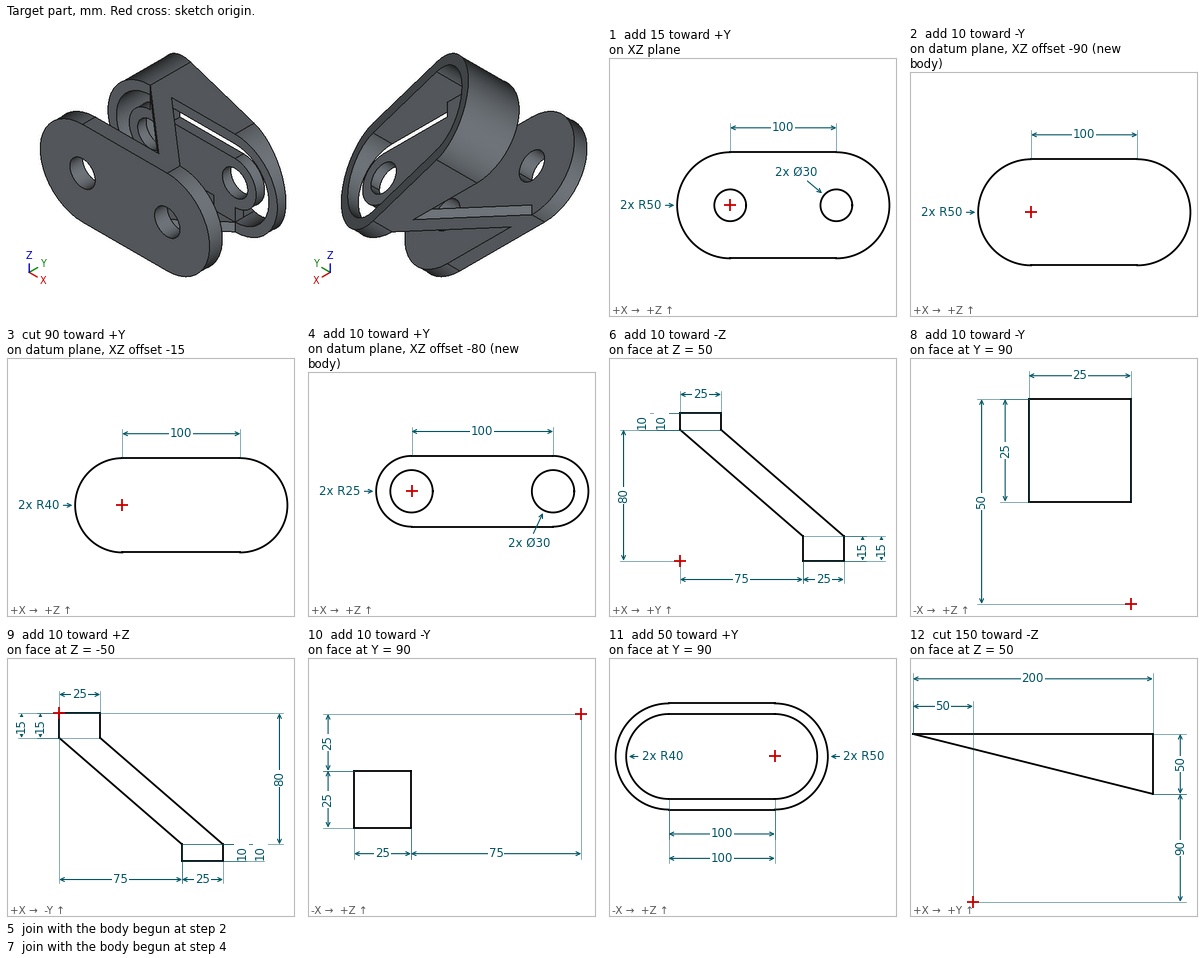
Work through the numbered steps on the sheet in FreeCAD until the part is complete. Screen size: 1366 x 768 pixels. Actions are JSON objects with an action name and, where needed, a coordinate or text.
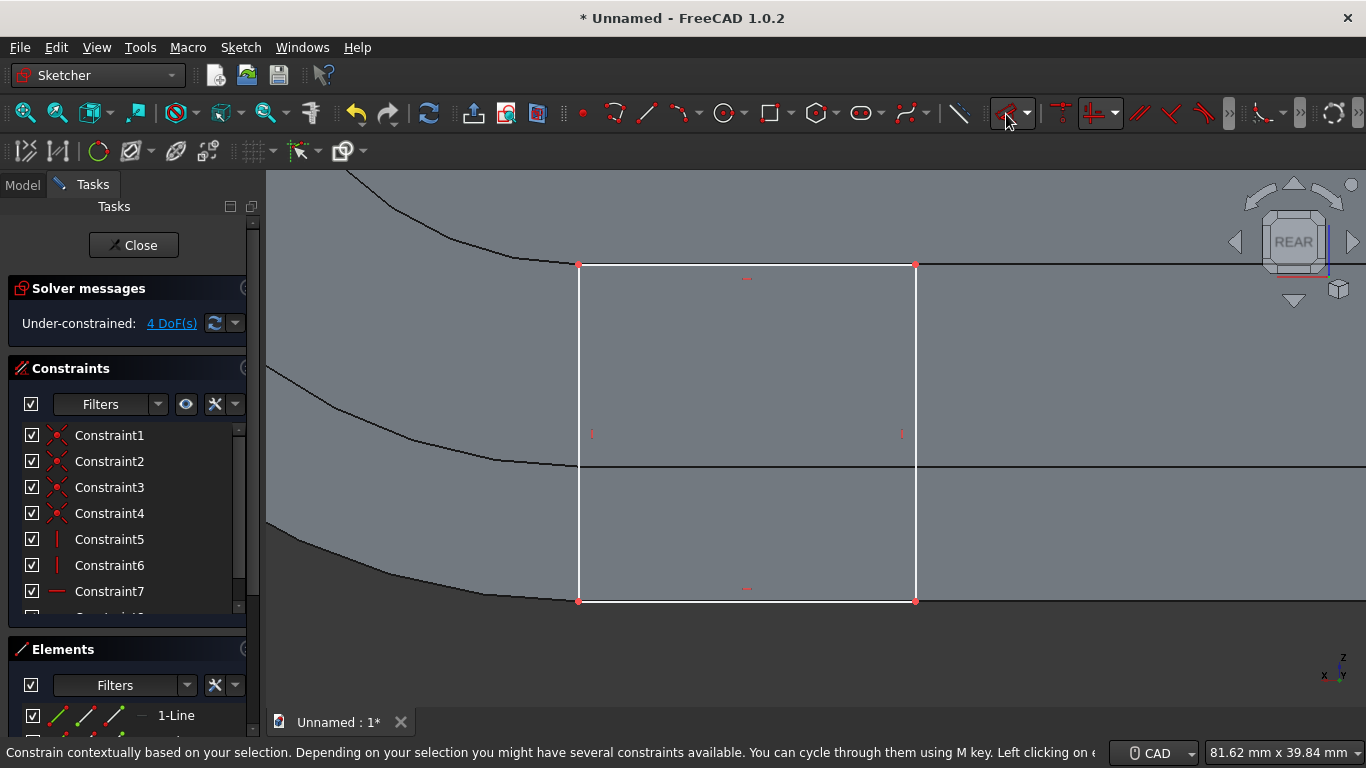
{"action": "left_click", "coordinate": [579, 366]}
{"action": "left_click", "coordinate": [545, 433]}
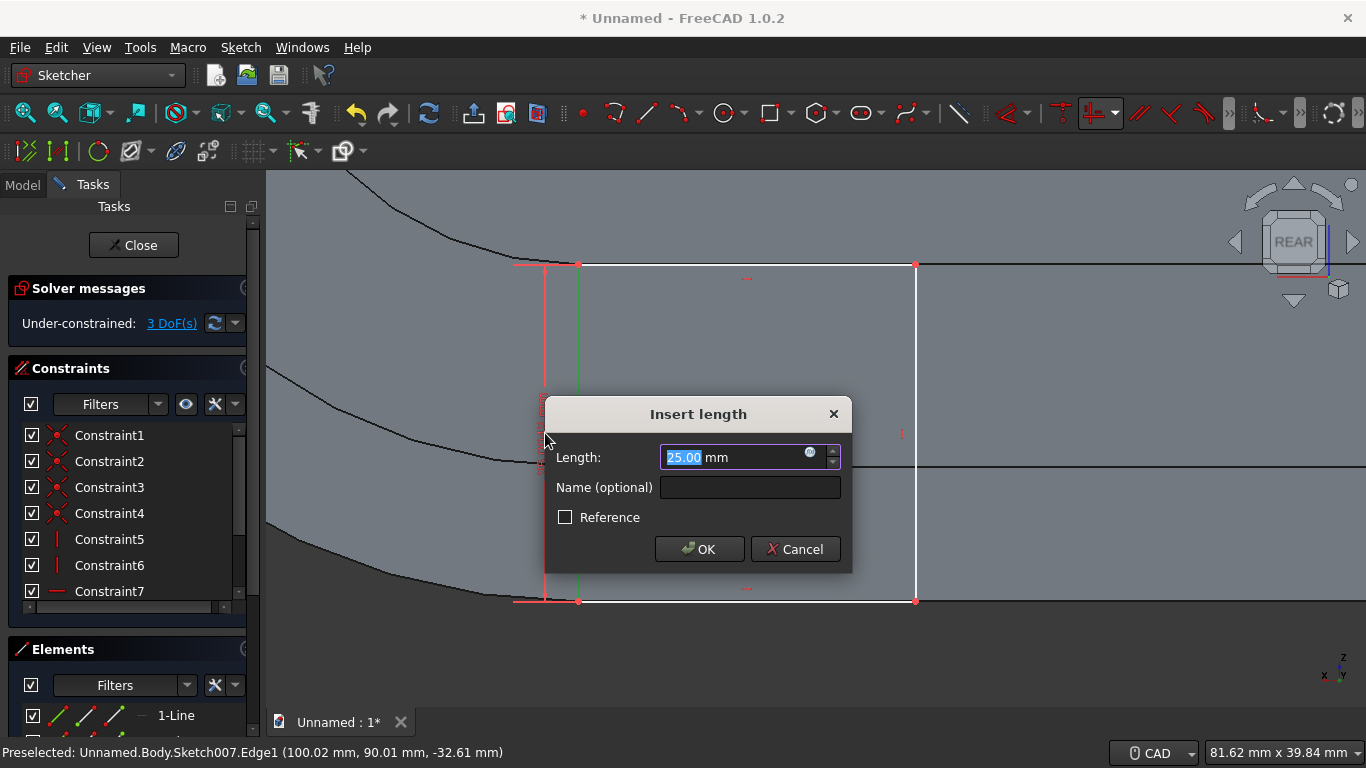
{"action": "type", "text": "25"}
{"action": "key", "text": "Return"}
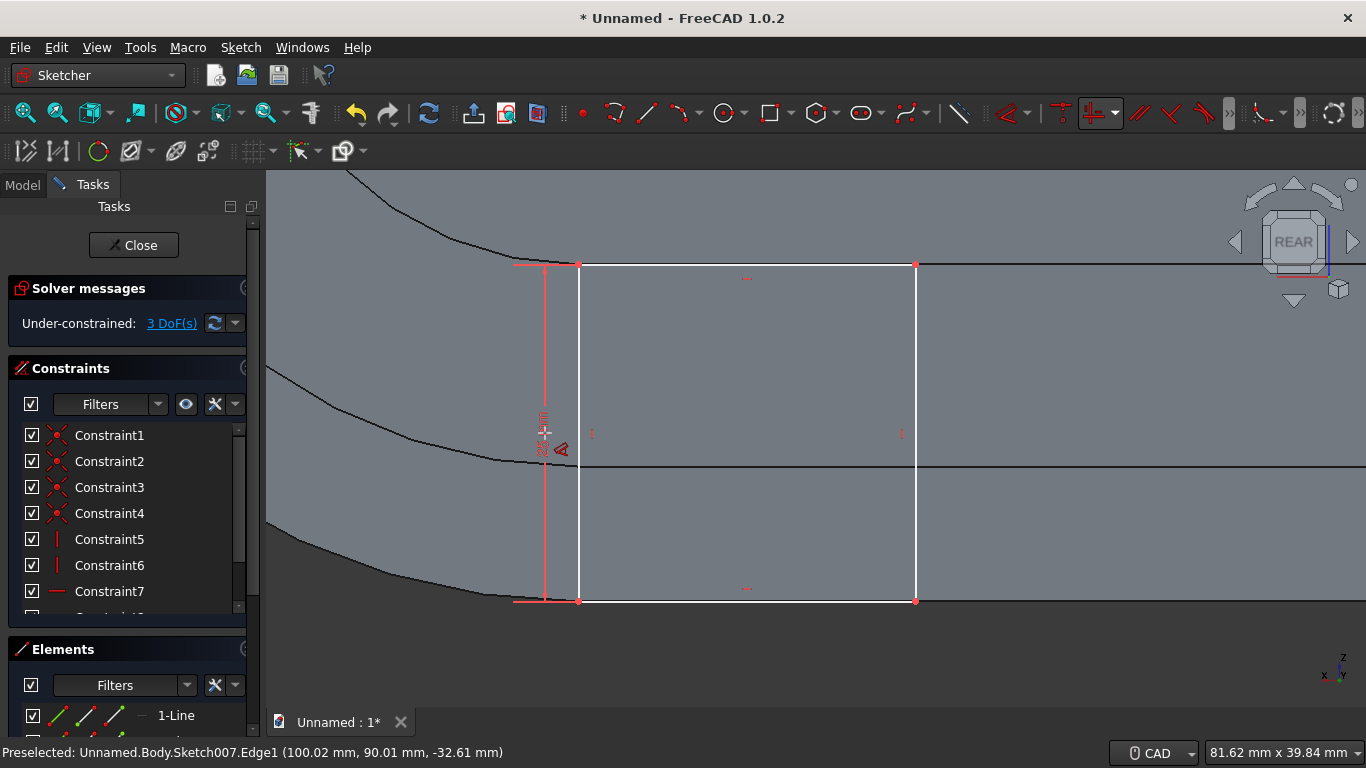
{"action": "left_click", "coordinate": [680, 602]}
{"action": "left_click", "coordinate": [747, 636]}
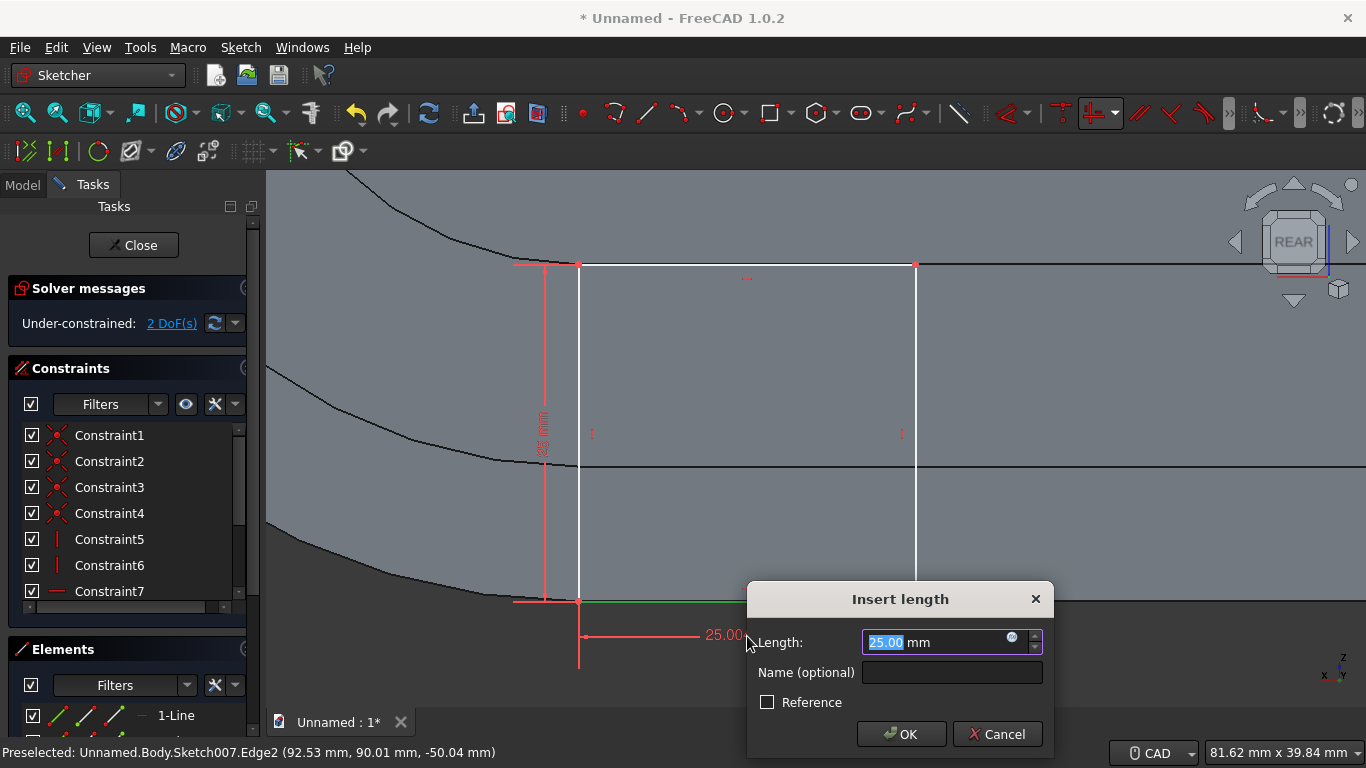
{"action": "type", "text": "25"}
{"action": "key", "text": "Return"}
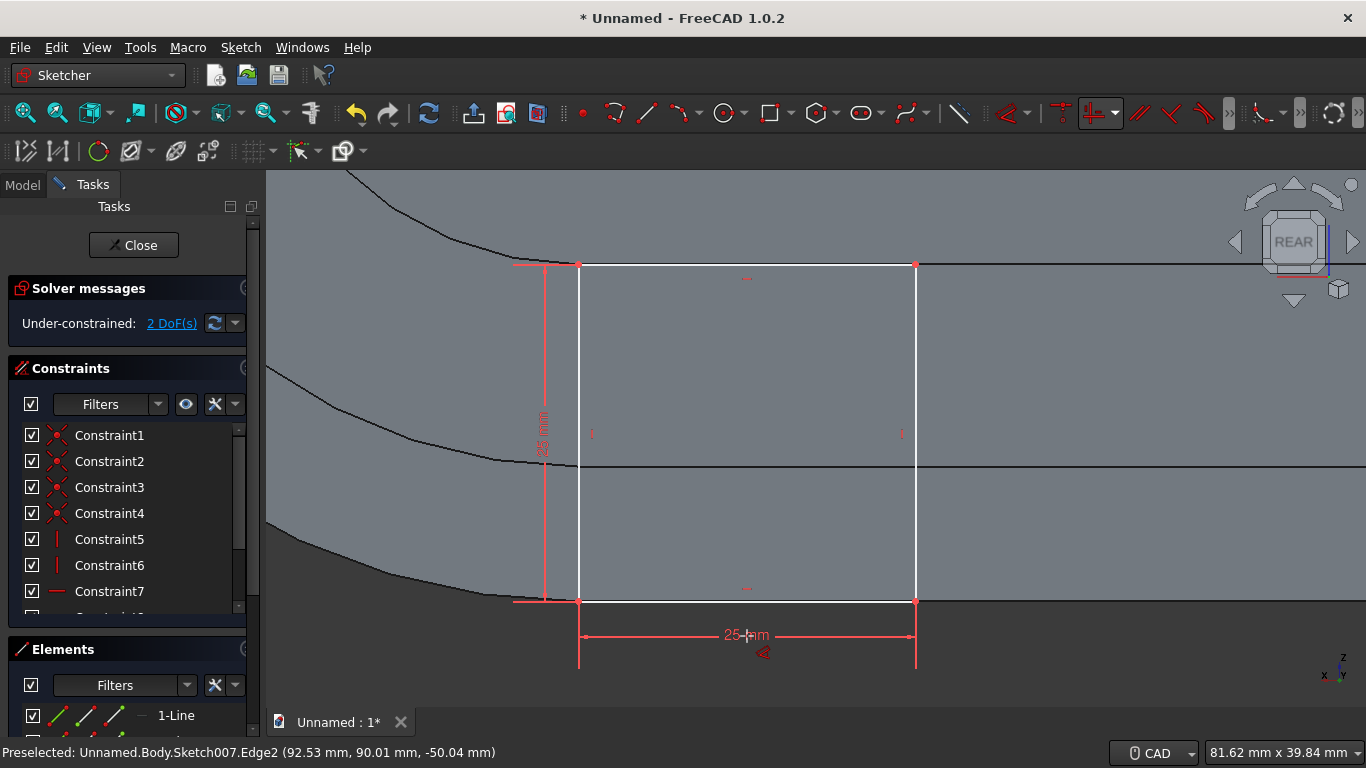
{"action": "left_click", "coordinate": [579, 265]}
{"action": "left_click", "coordinate": [545, 231]}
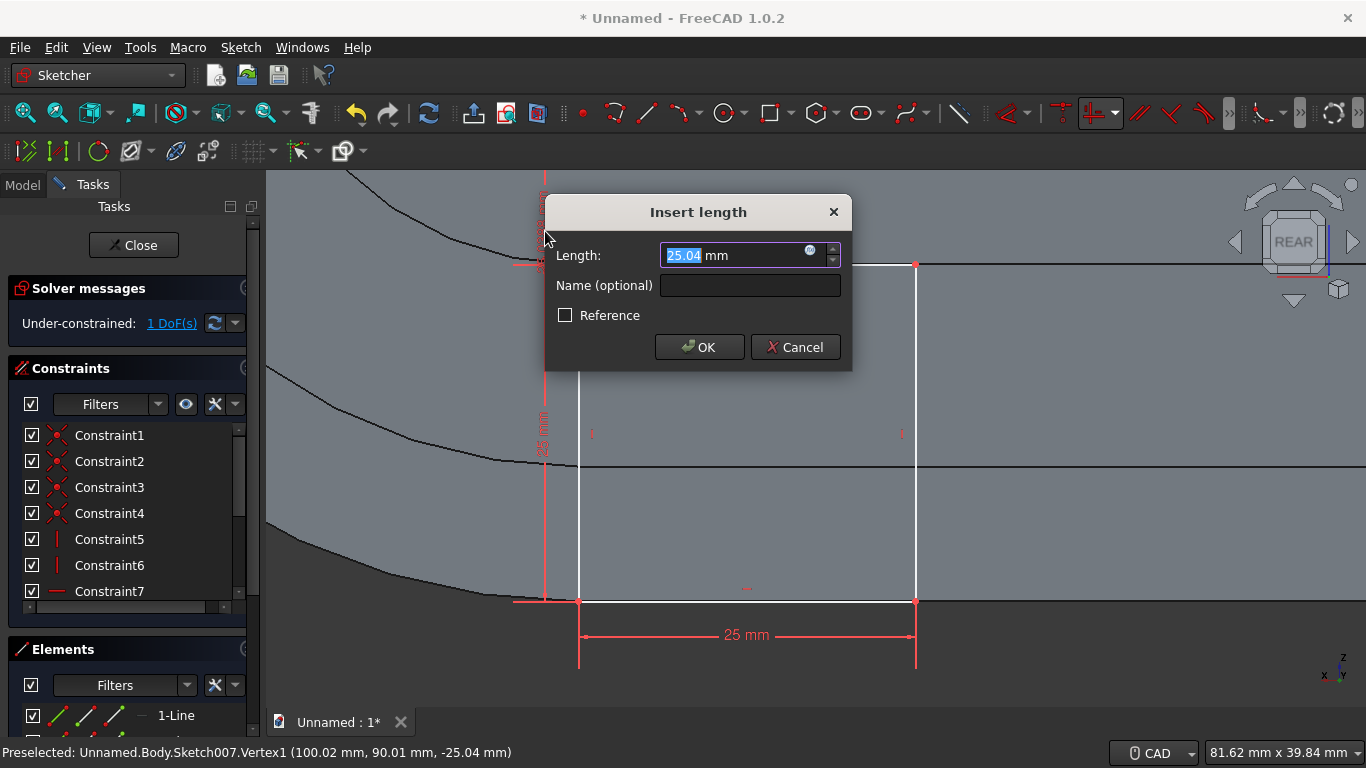
{"action": "type", "text": "25"}
{"action": "key", "text": "Return"}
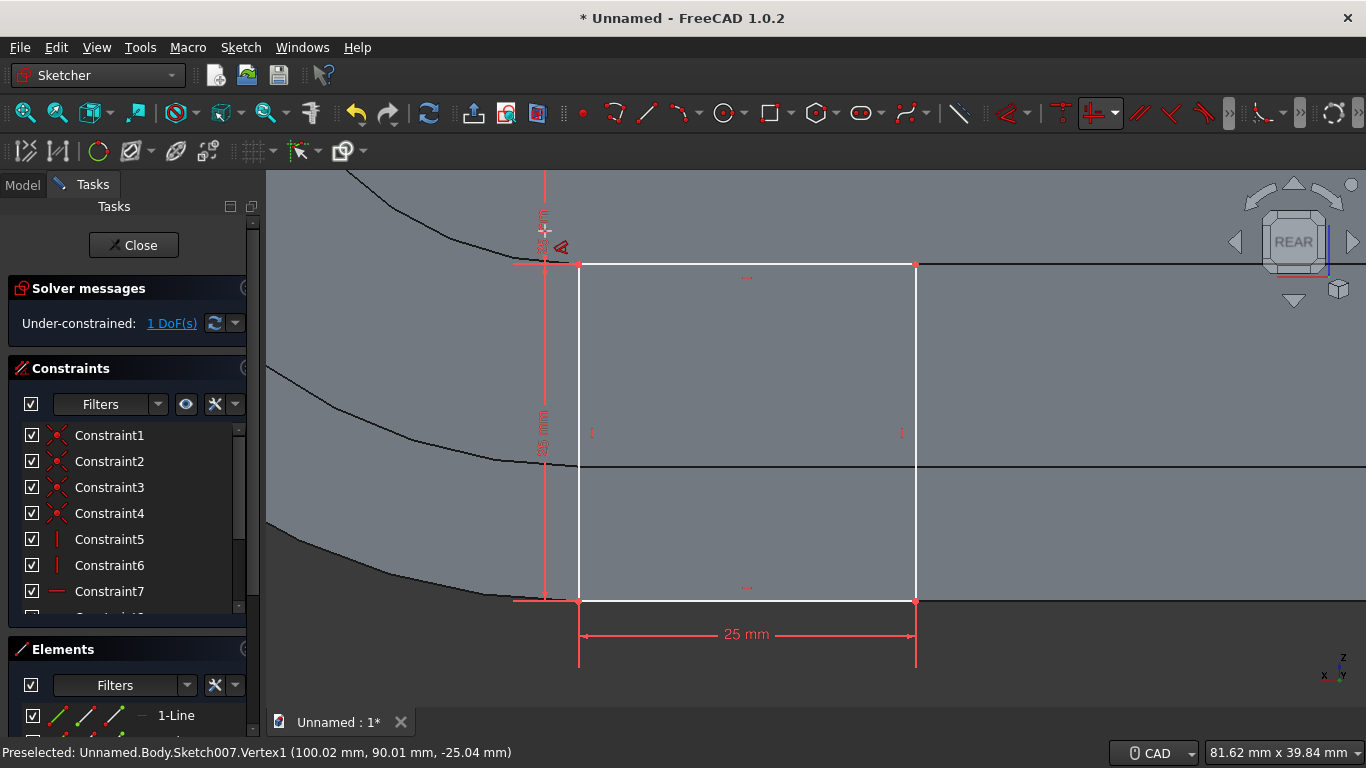
{"action": "left_click", "coordinate": [916, 601]}
{"action": "left_click", "coordinate": [1058, 635]}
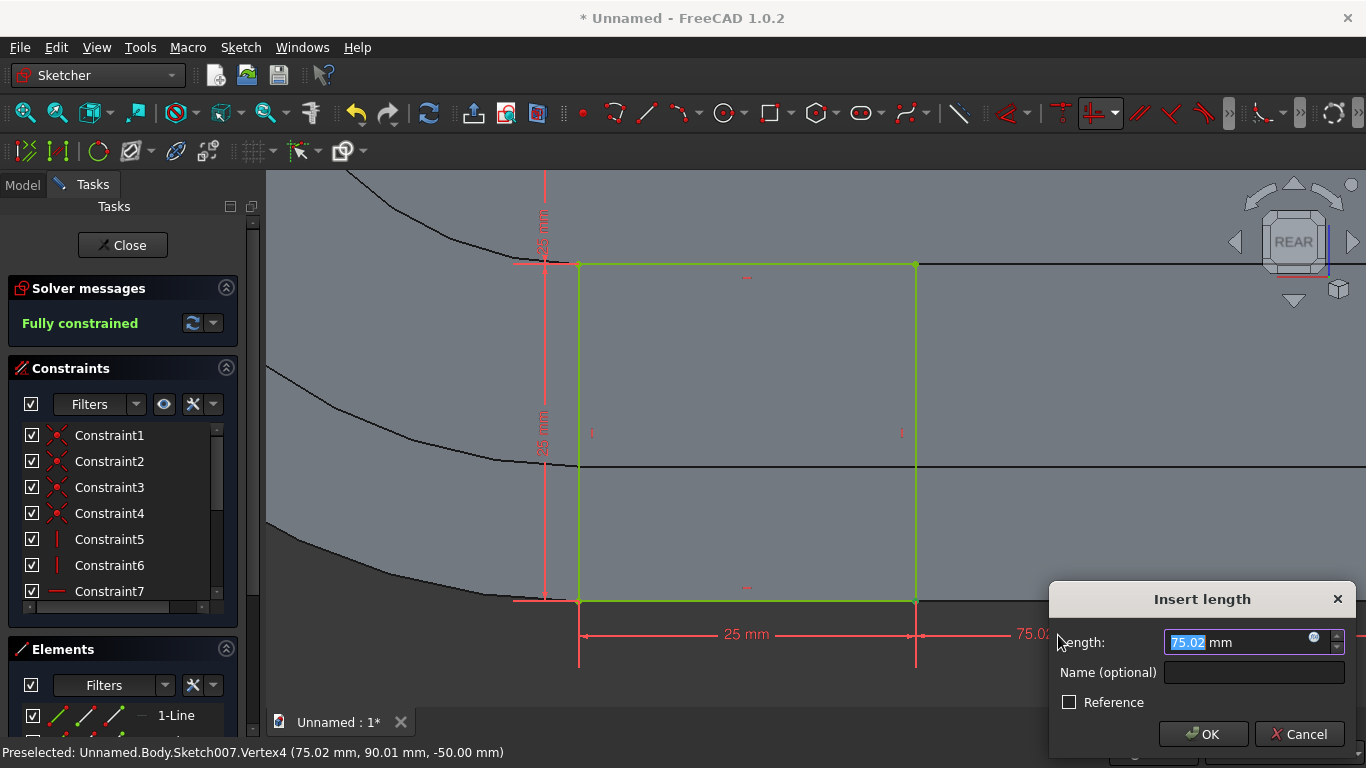
{"action": "type", "text": "75"}
{"action": "key", "text": "Return"}
{"action": "key", "text": "Escape"}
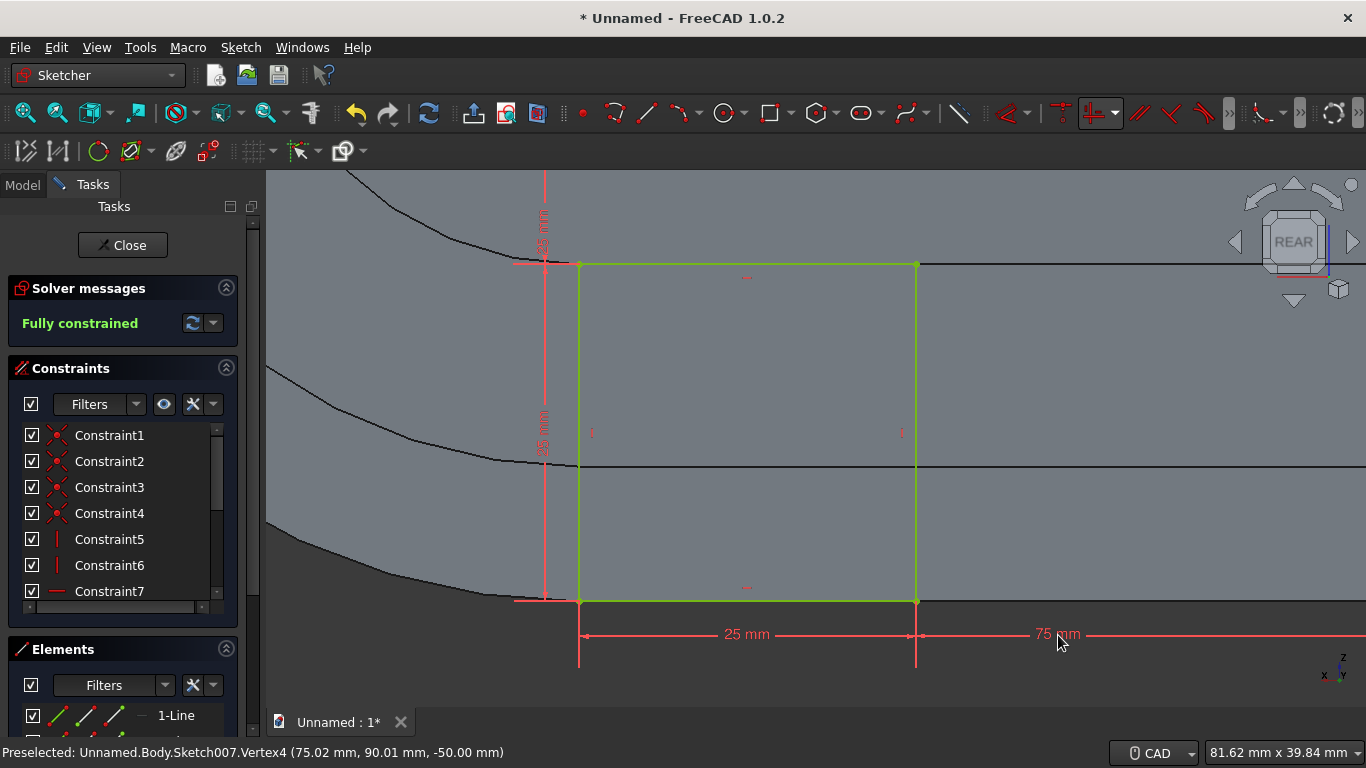
{"action": "left_click", "coordinate": [123, 245]}